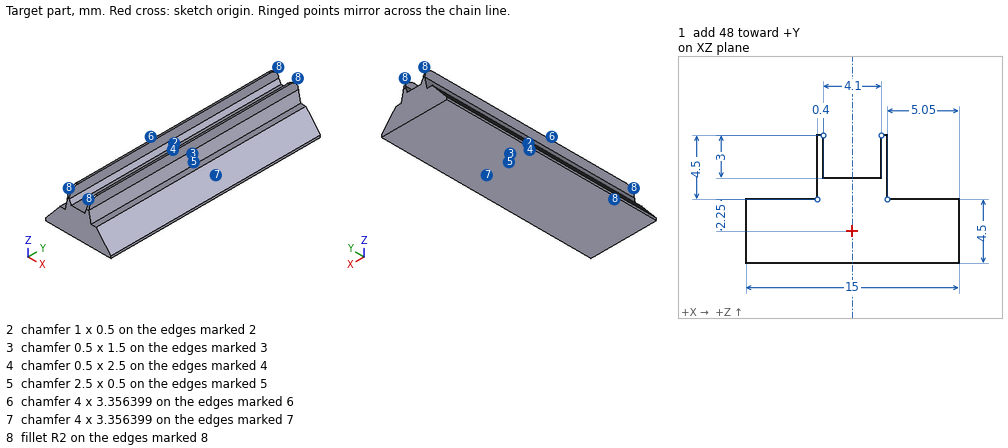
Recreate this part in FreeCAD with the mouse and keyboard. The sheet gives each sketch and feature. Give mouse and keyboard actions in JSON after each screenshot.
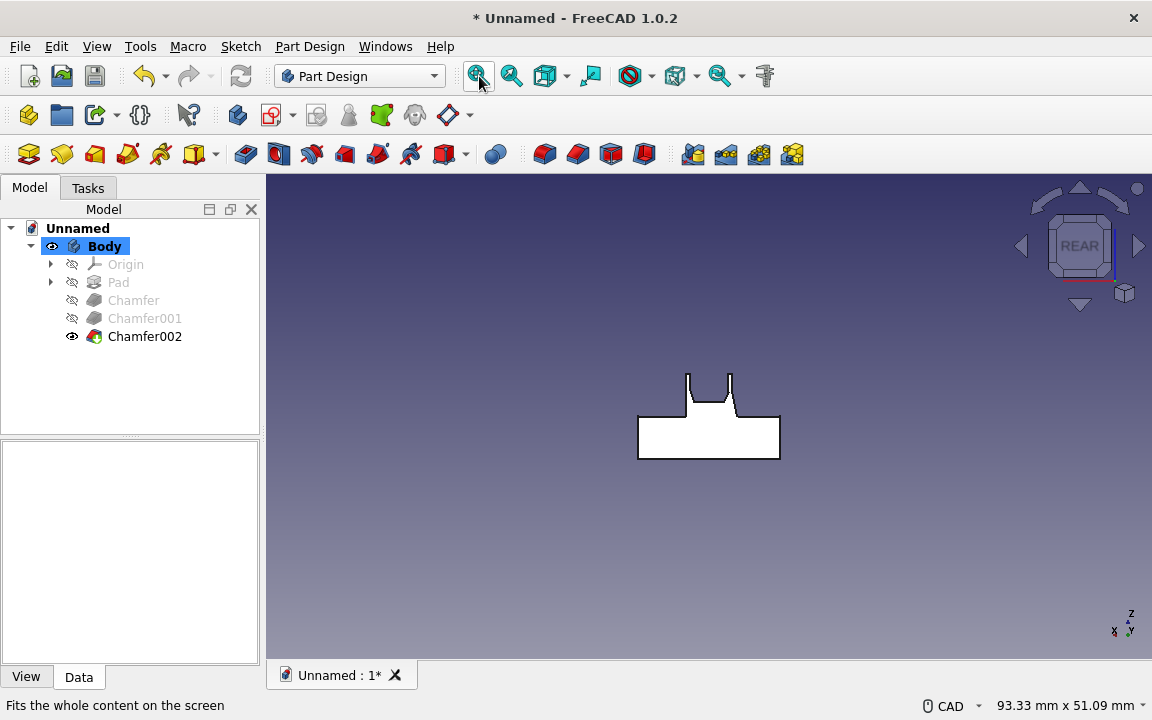
{"action": "key", "text": "6"}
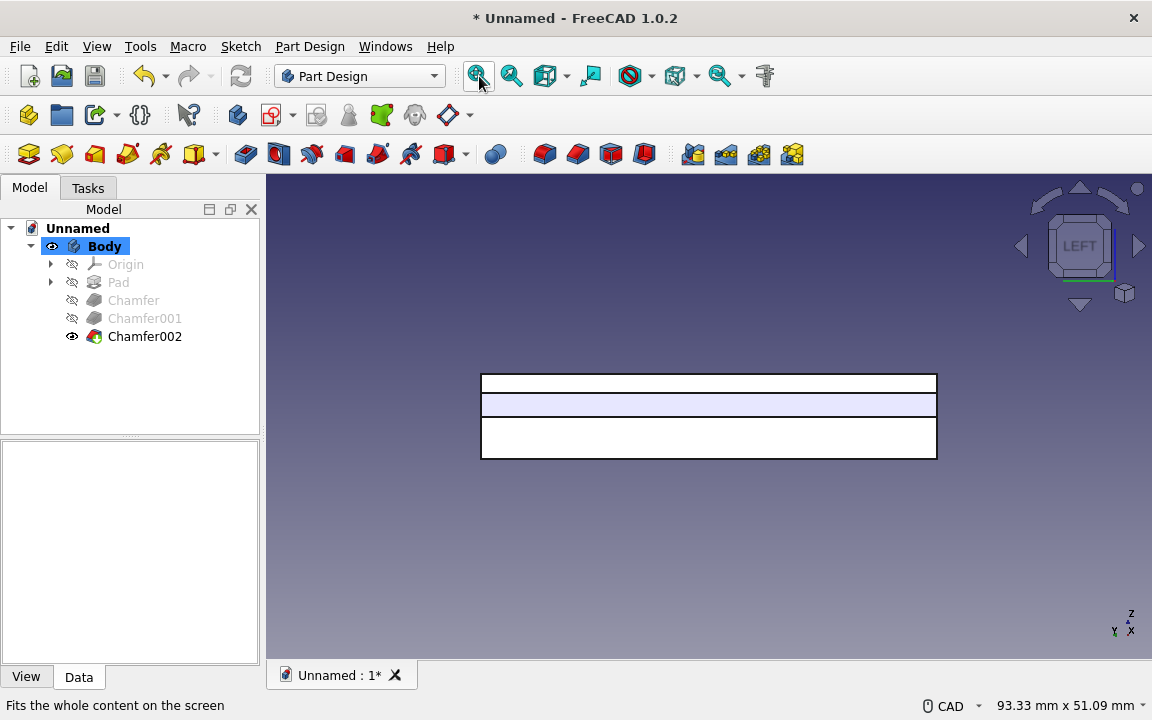
{"action": "key", "text": "v 3"}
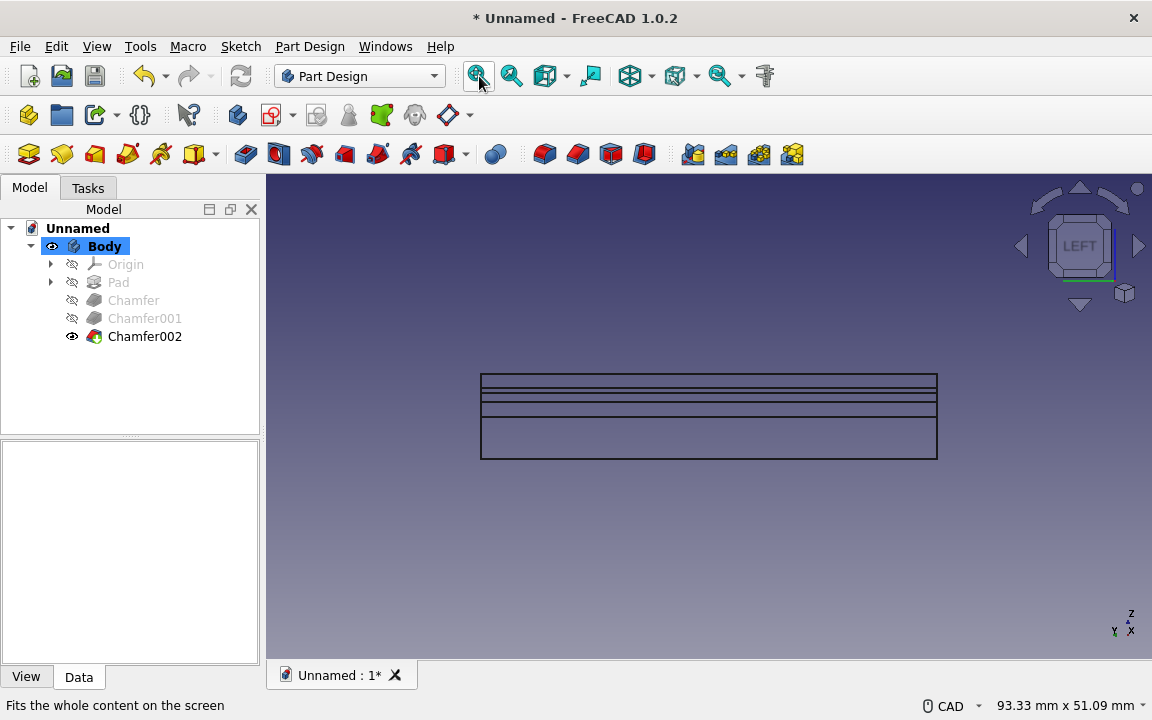
{"action": "key", "text": "0"}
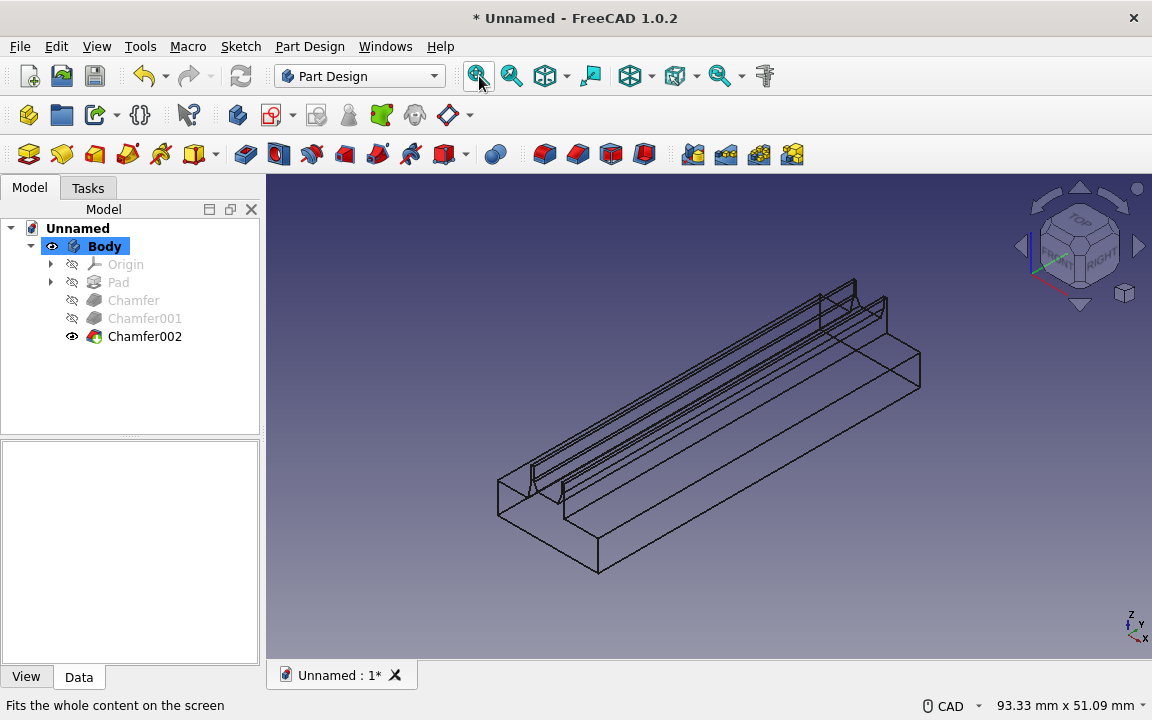
{"action": "left_click", "coordinate": [725, 425]}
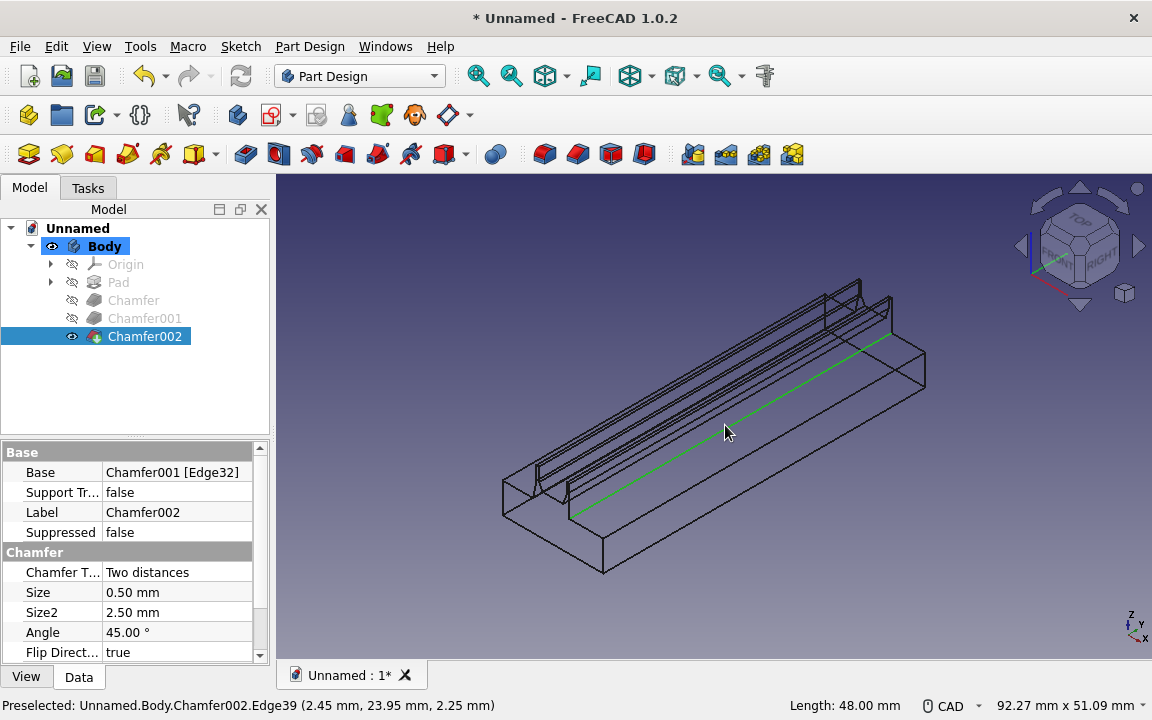
{"action": "key", "text": "v 1"}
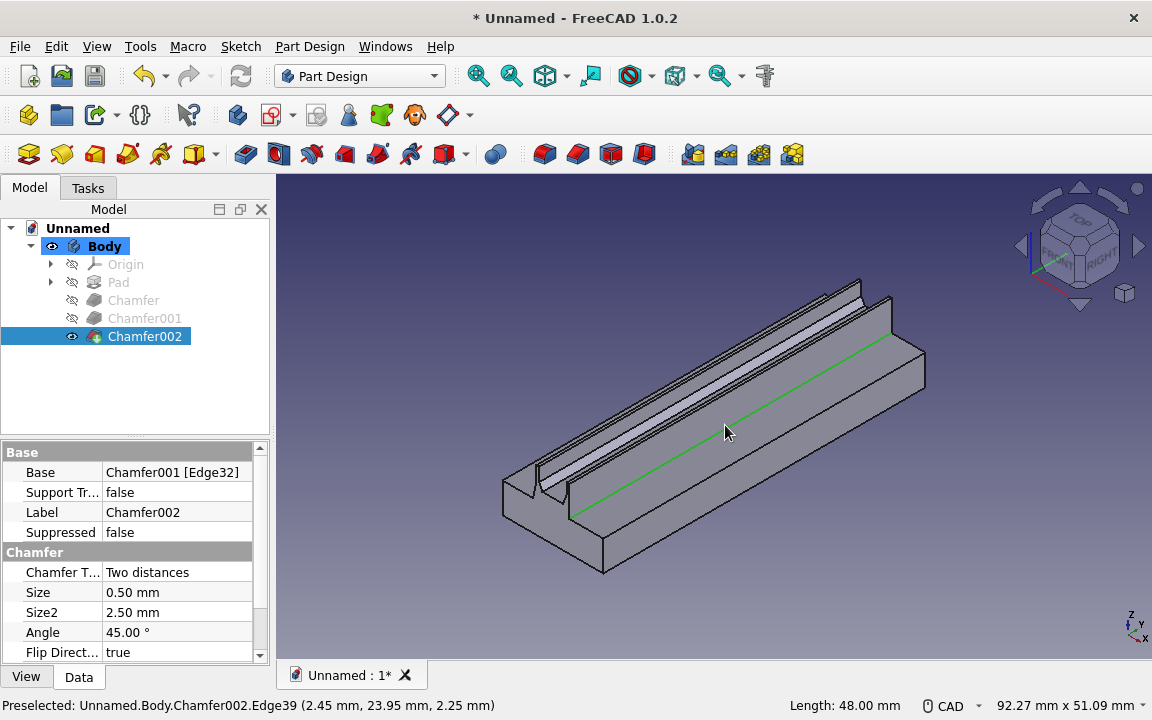
{"action": "left_click", "coordinate": [578, 154]}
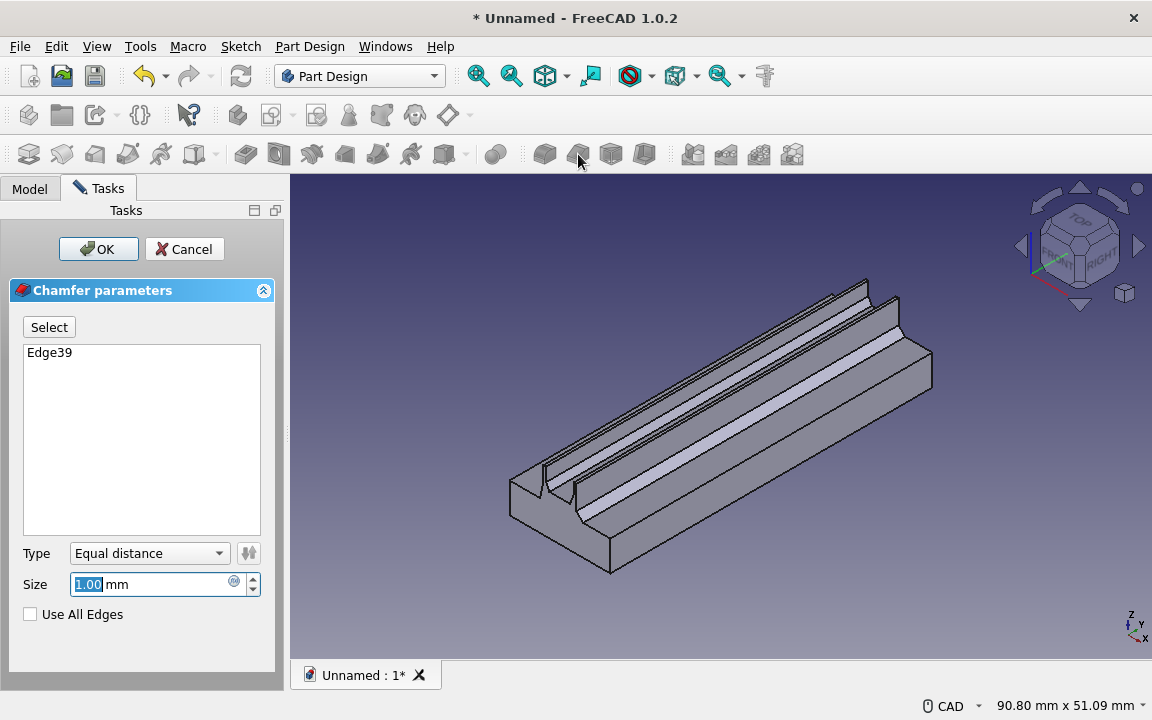
{"action": "type", "text": "2.5"}
{"action": "key", "text": "Tab"}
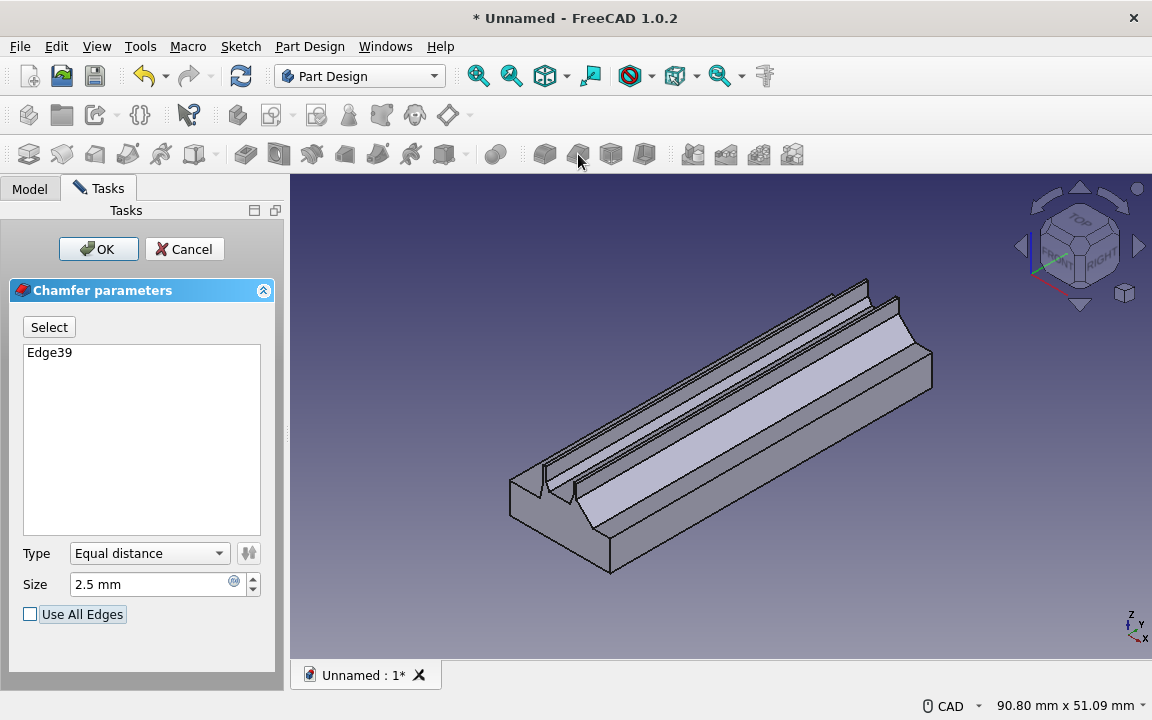
{"action": "left_click", "coordinate": [150, 554]}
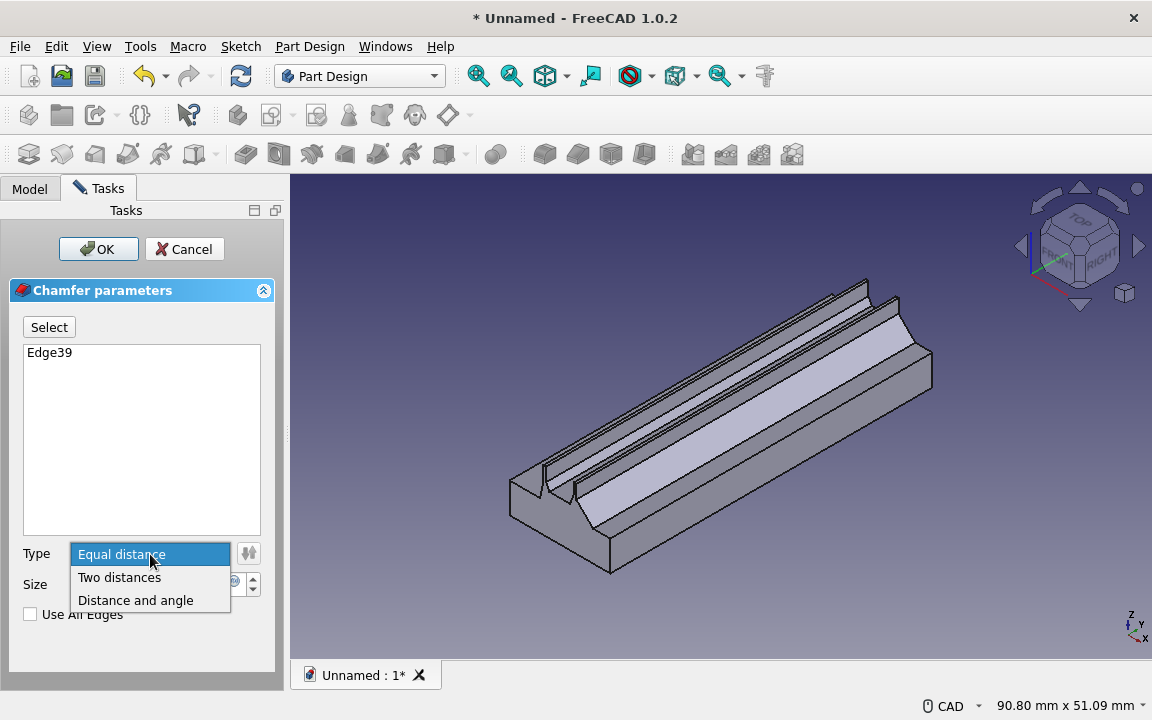
{"action": "left_click", "coordinate": [148, 578]}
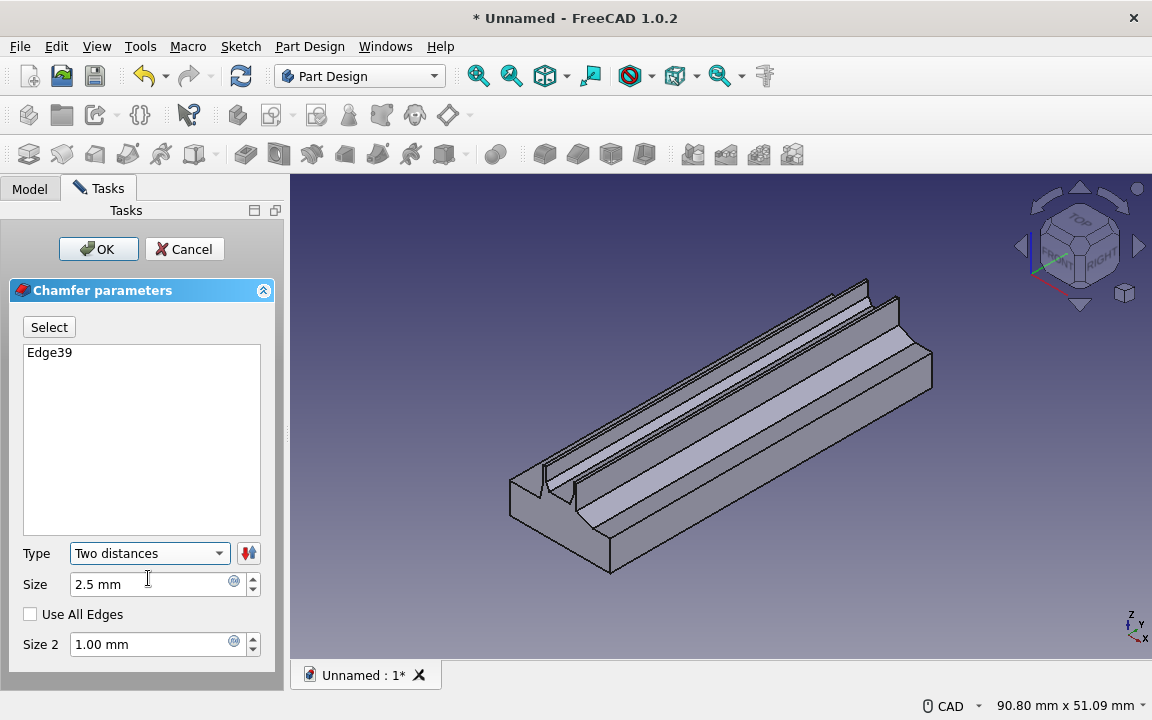
{"action": "triple_click", "coordinate": [158, 644]}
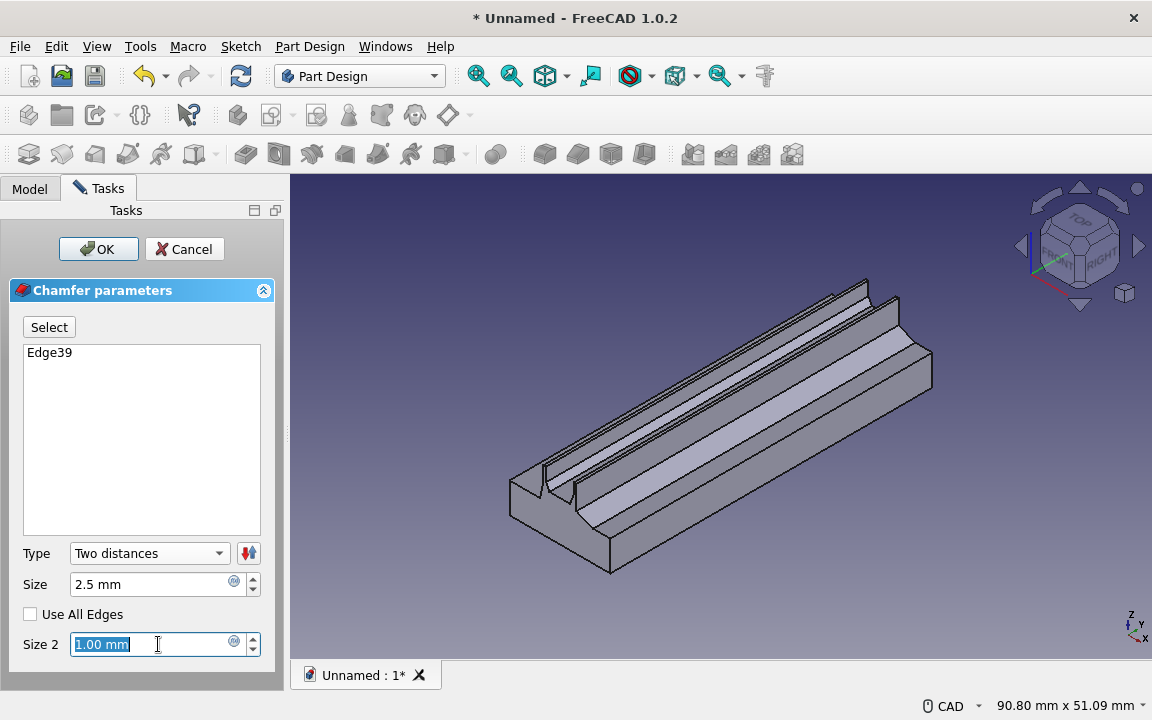
{"action": "type", "text": "0.5"}
{"action": "key", "text": "Tab"}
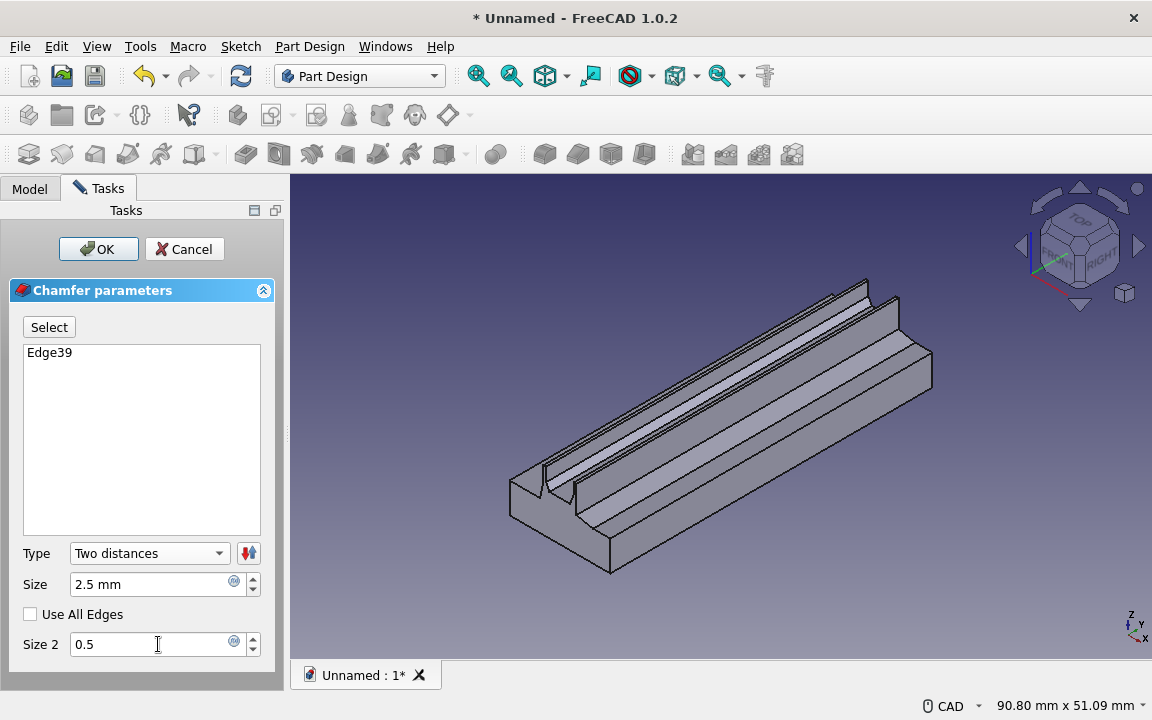
{"action": "left_click", "coordinate": [249, 554]}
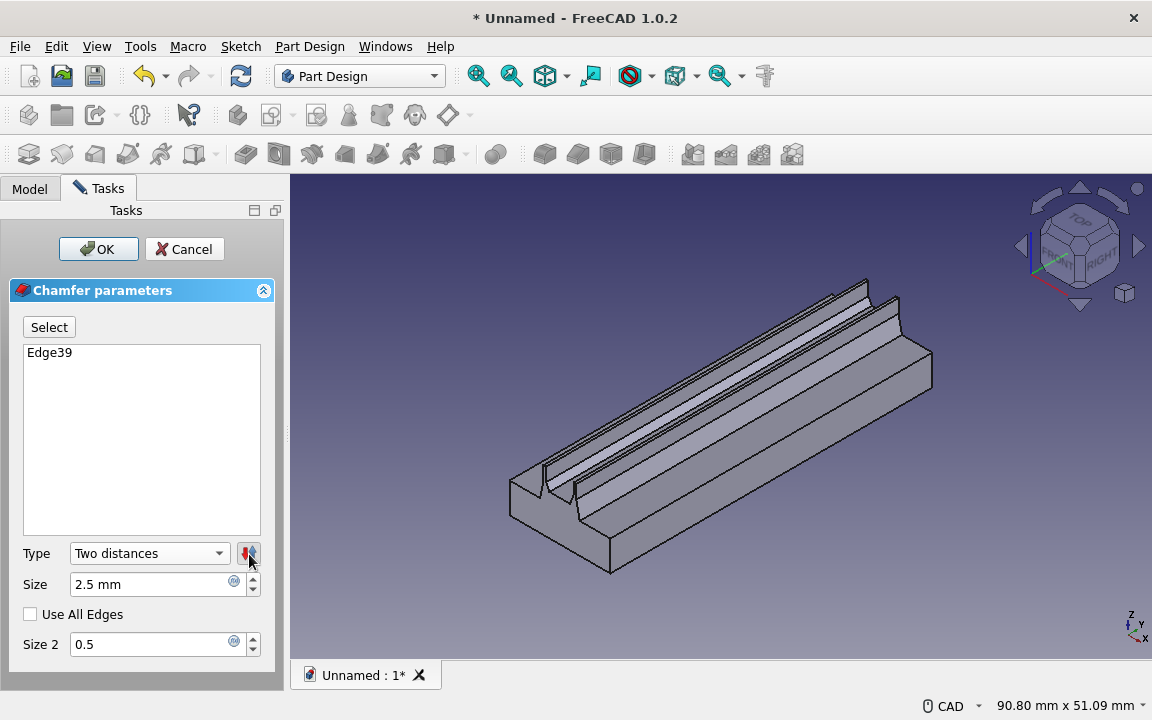
{"action": "left_click", "coordinate": [99, 249]}